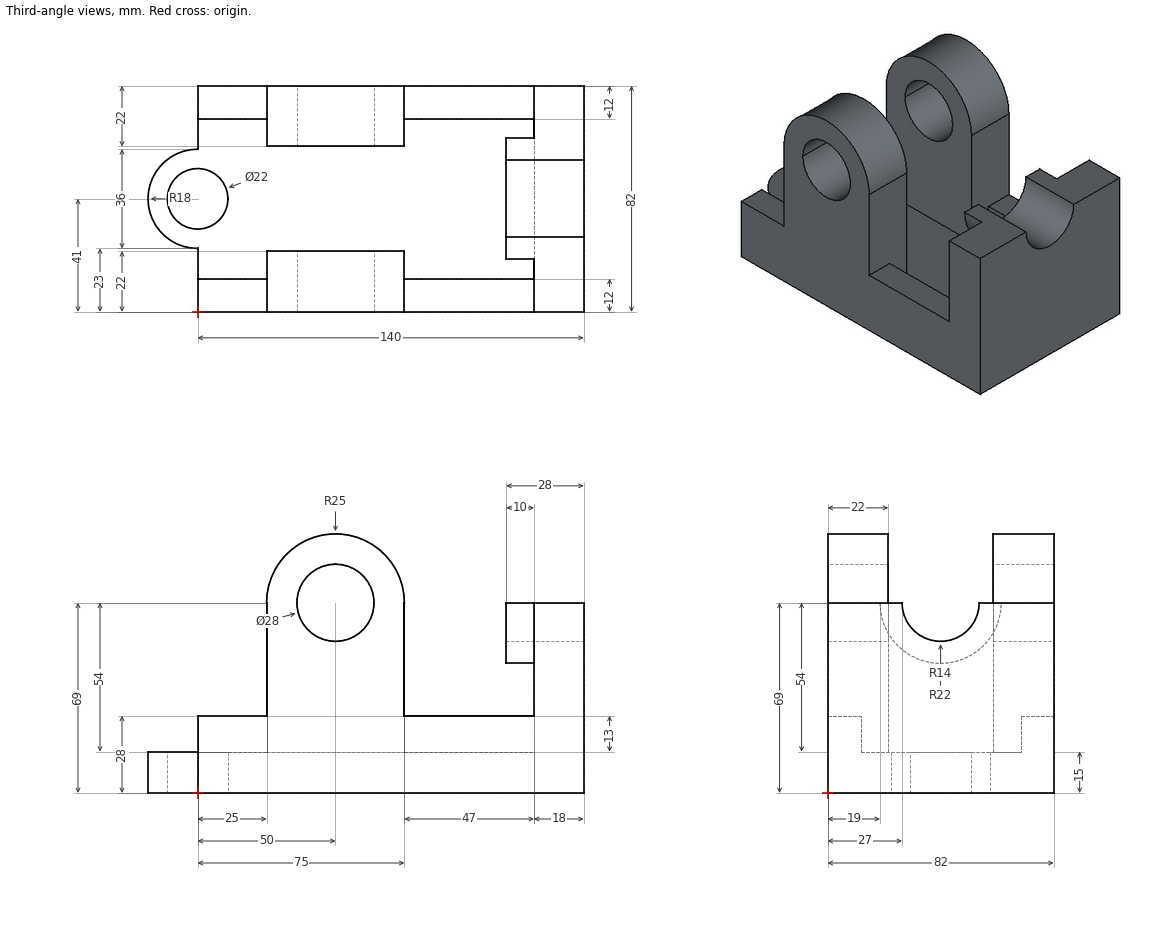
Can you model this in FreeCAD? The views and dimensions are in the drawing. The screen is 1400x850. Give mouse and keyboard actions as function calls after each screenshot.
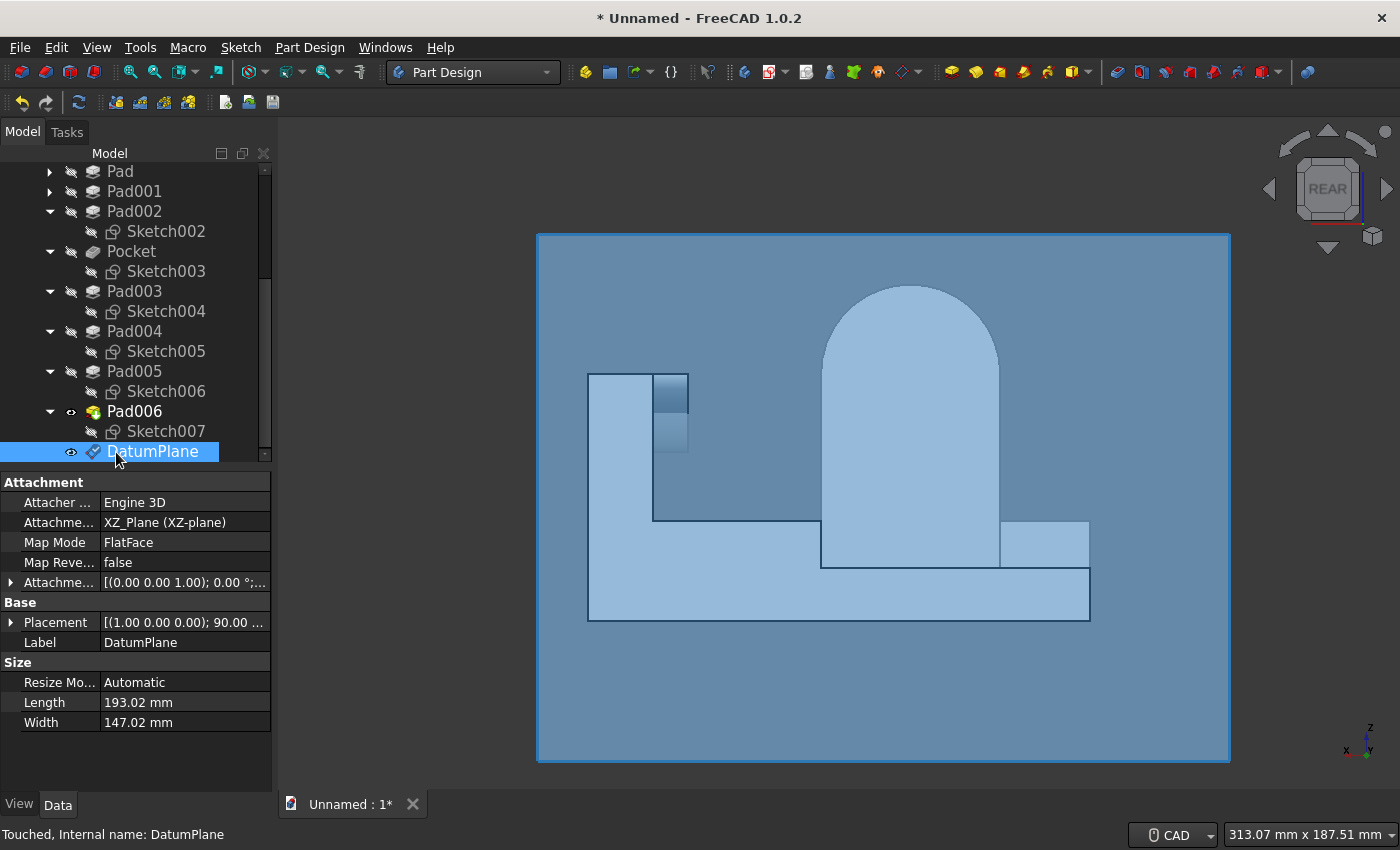
click(770, 72)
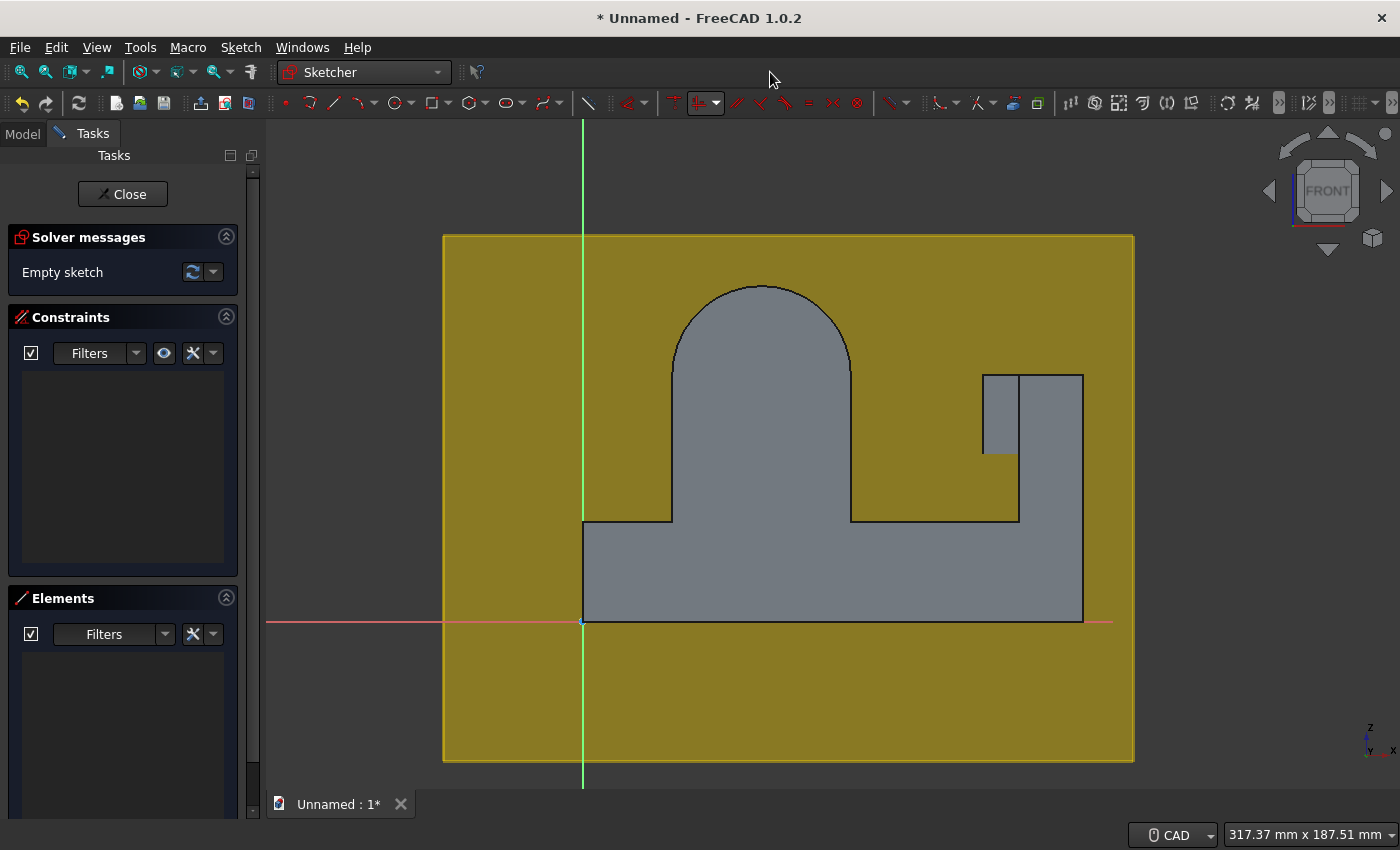
click(250, 104)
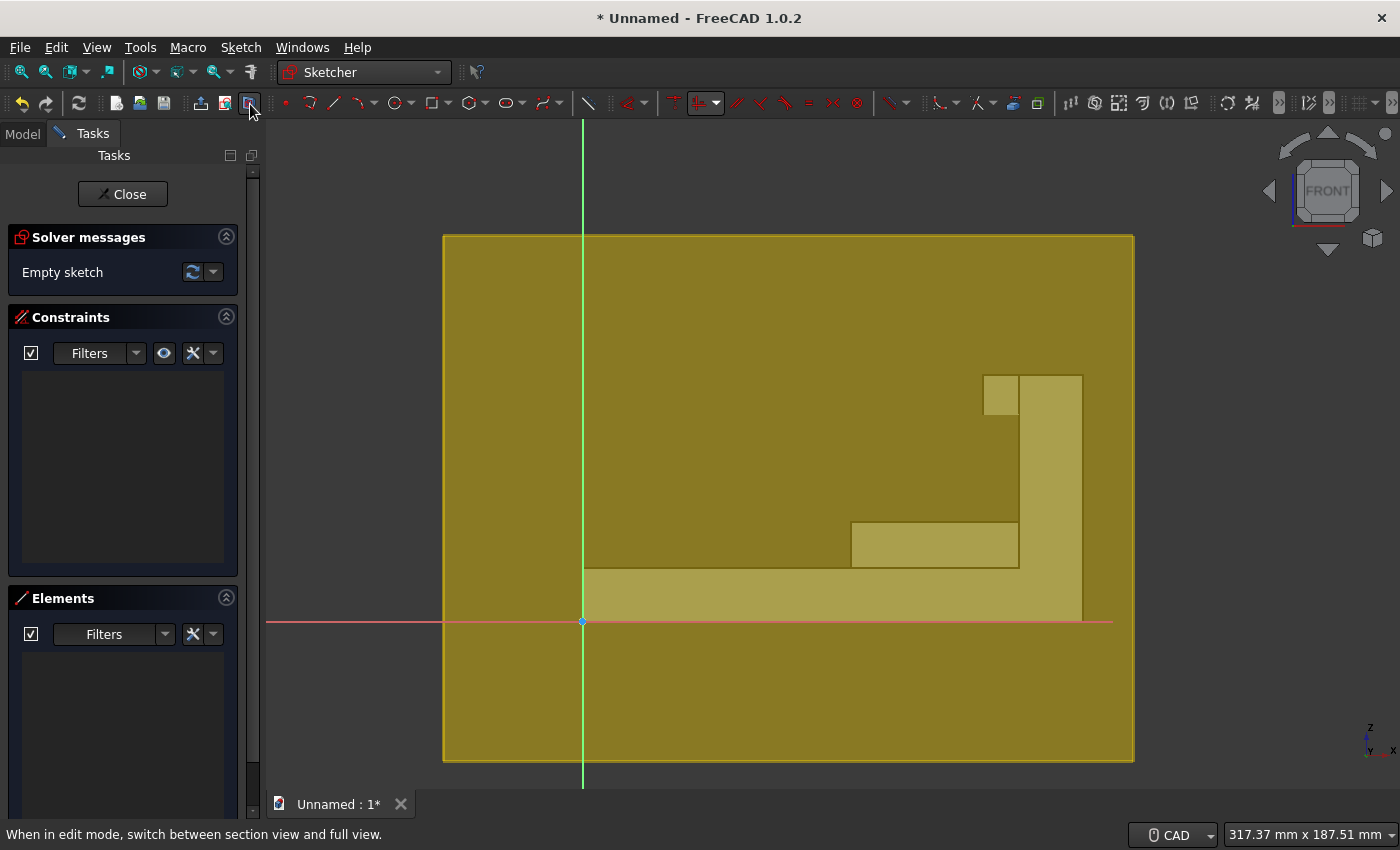
click(310, 104)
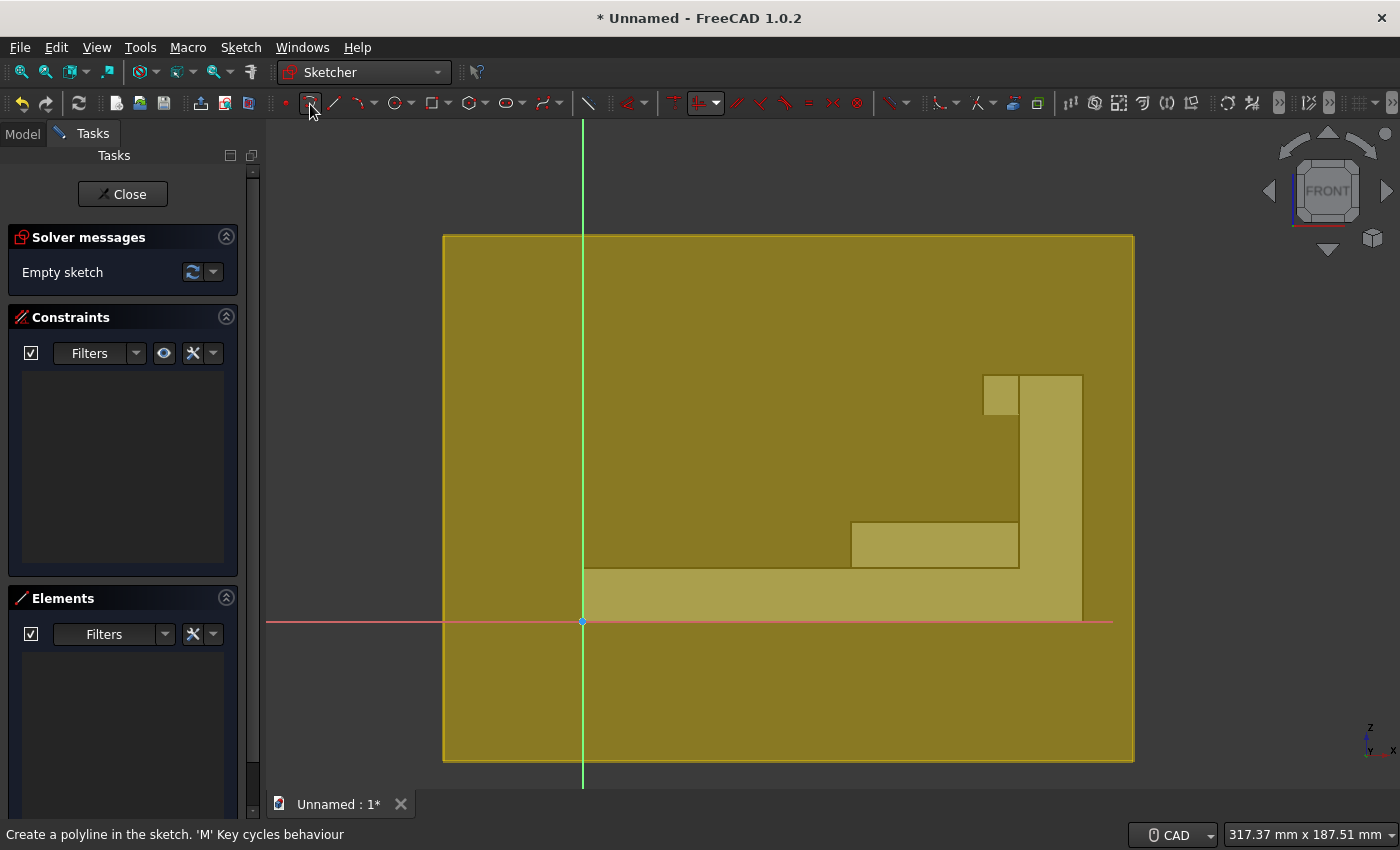
click(851, 375)
click(851, 568)
click(672, 568)
click(672, 375)
right_click(672, 375)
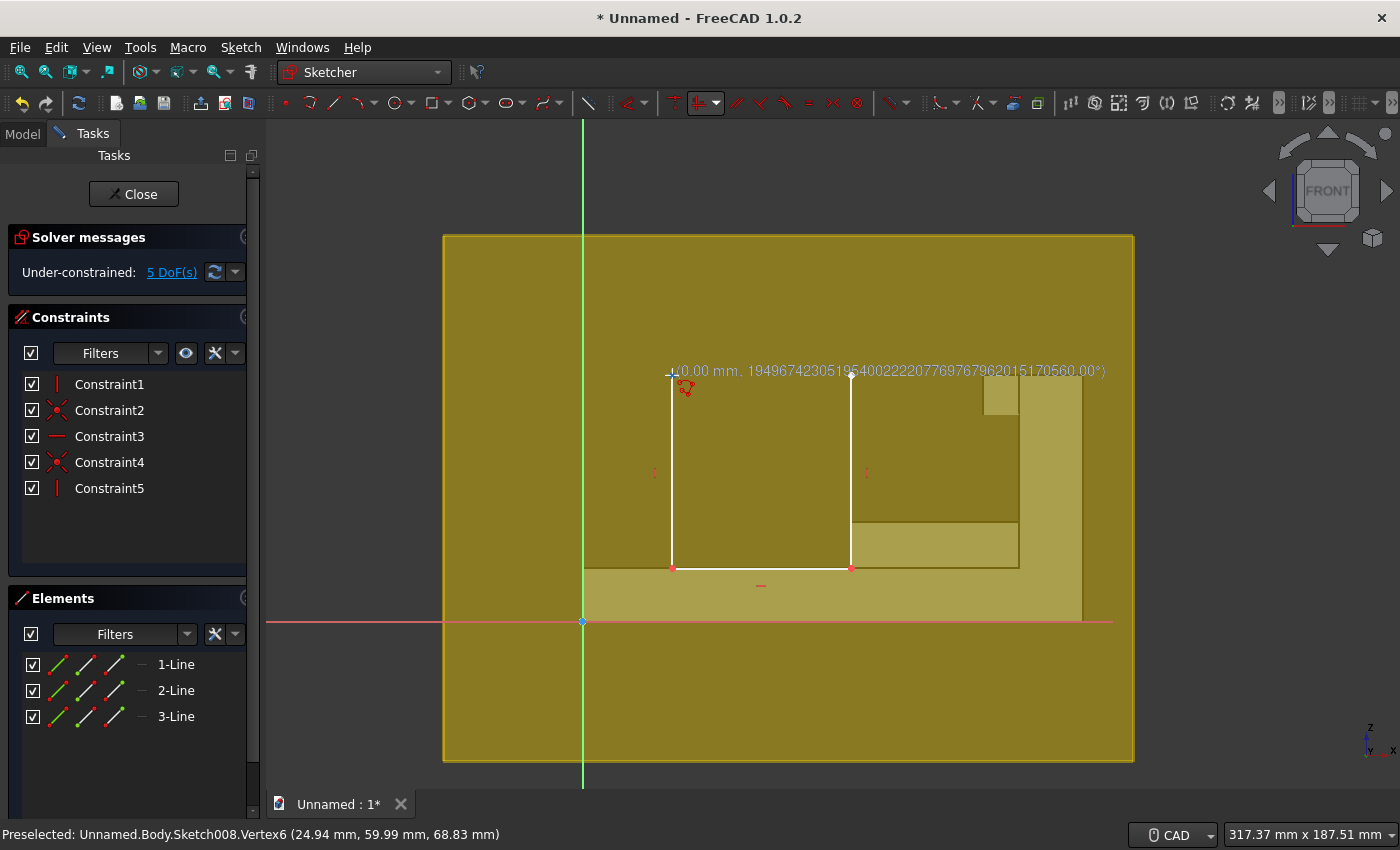
click(358, 104)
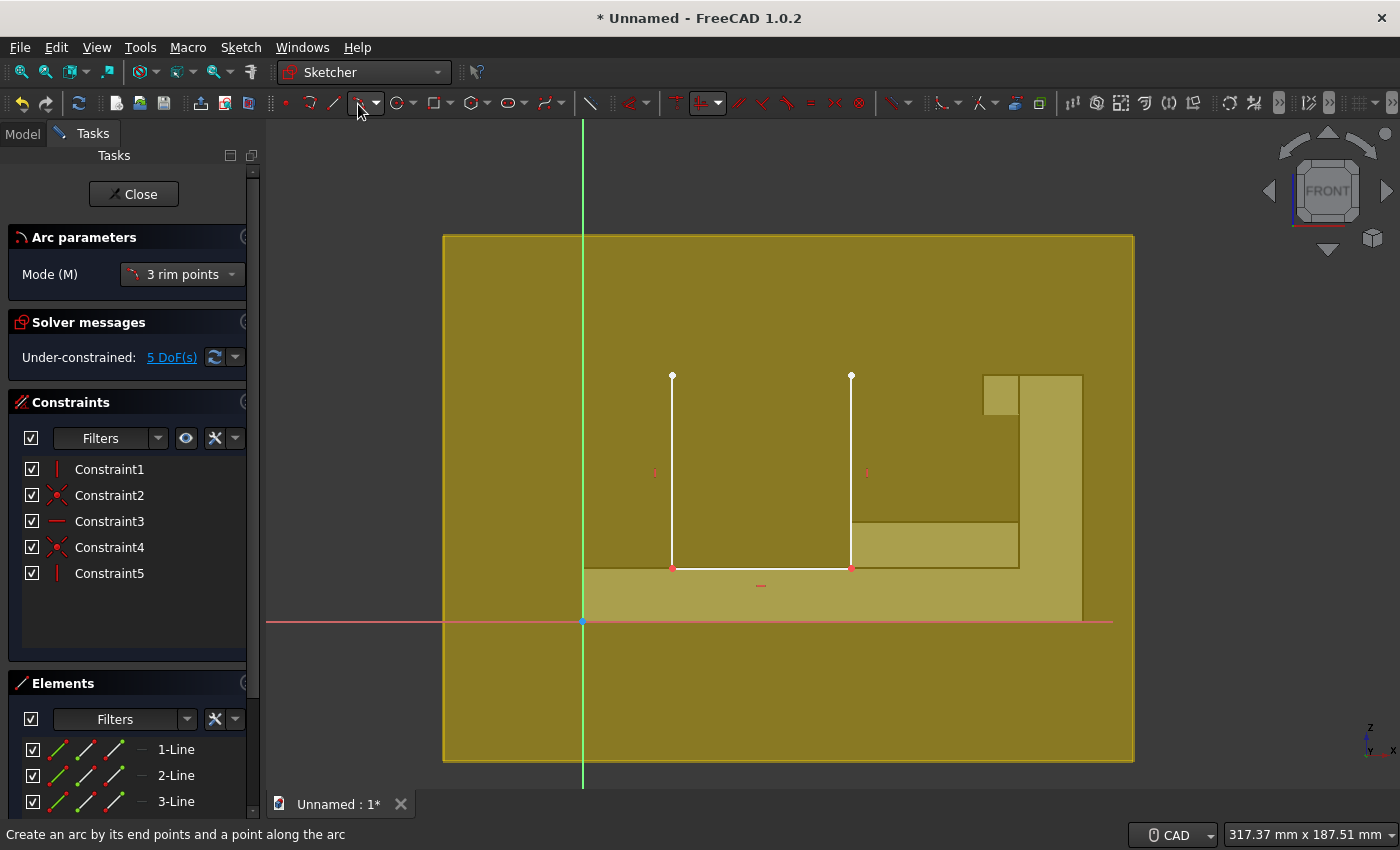
click(672, 376)
click(851, 376)
click(762, 286)
key(Escape)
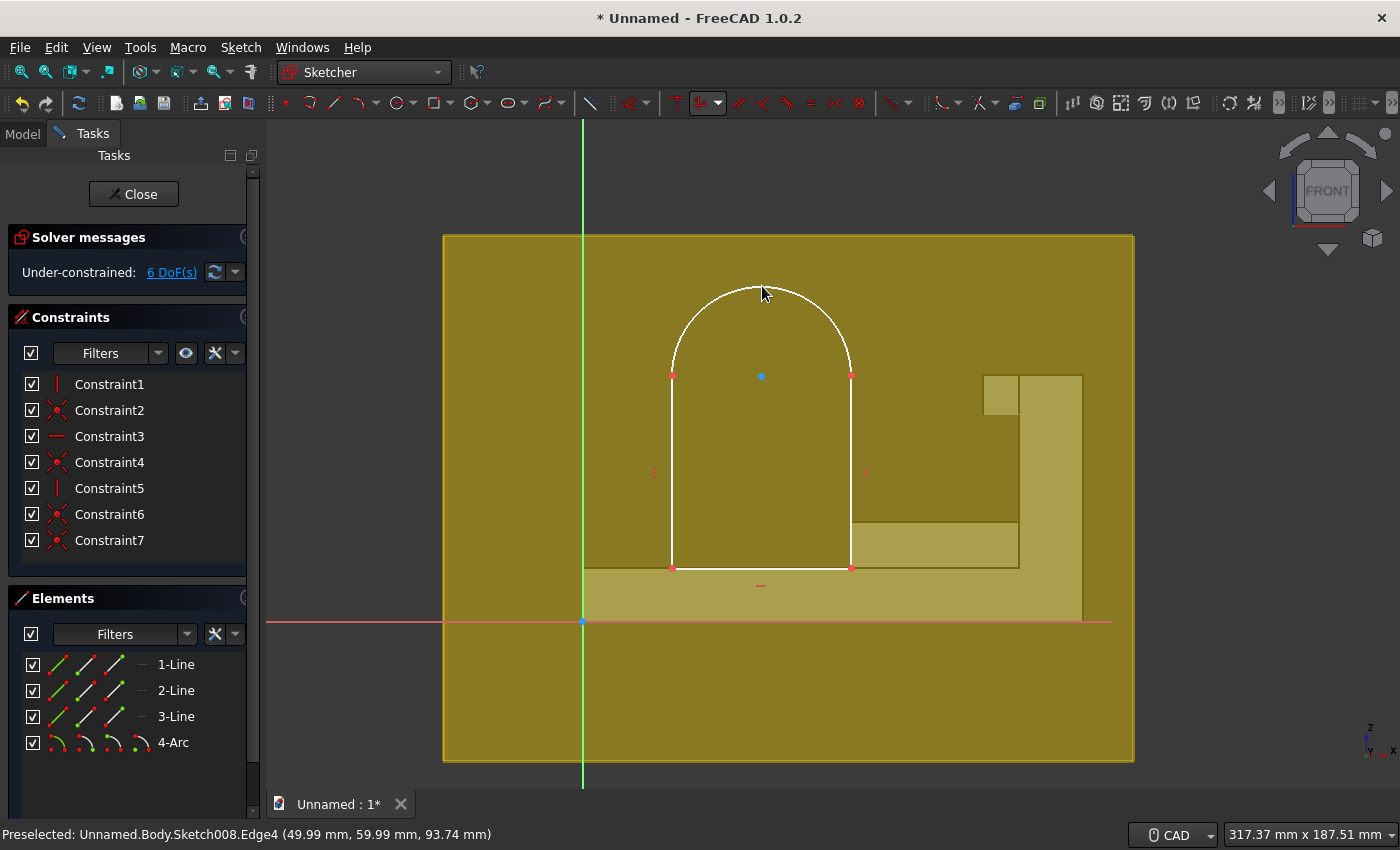
click(851, 434)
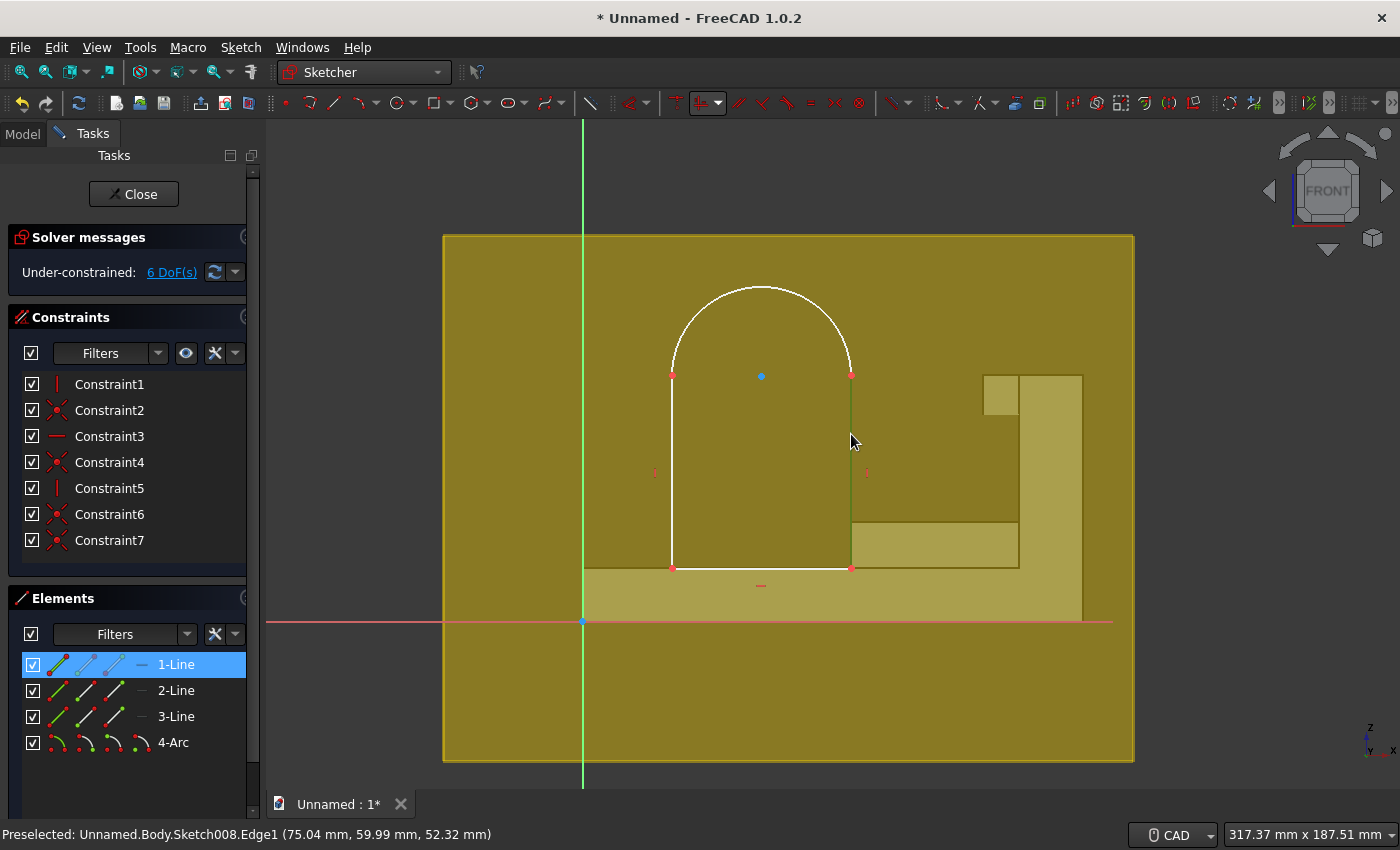
click(814, 304)